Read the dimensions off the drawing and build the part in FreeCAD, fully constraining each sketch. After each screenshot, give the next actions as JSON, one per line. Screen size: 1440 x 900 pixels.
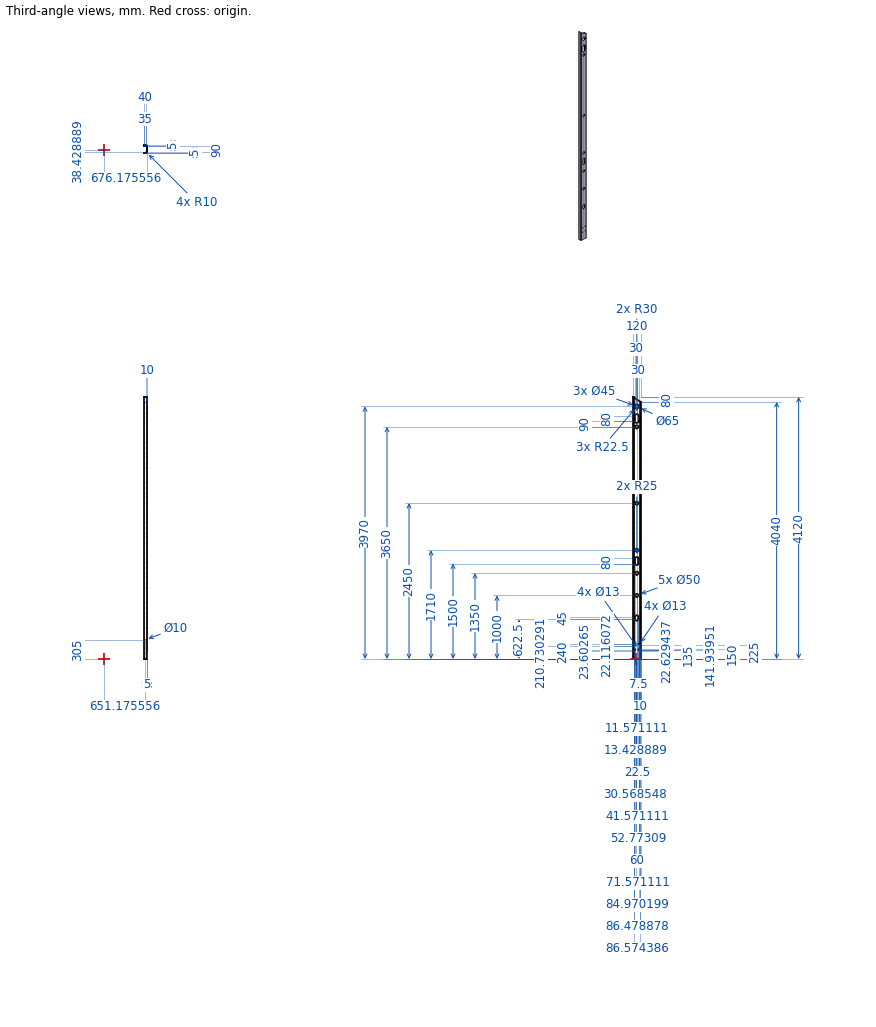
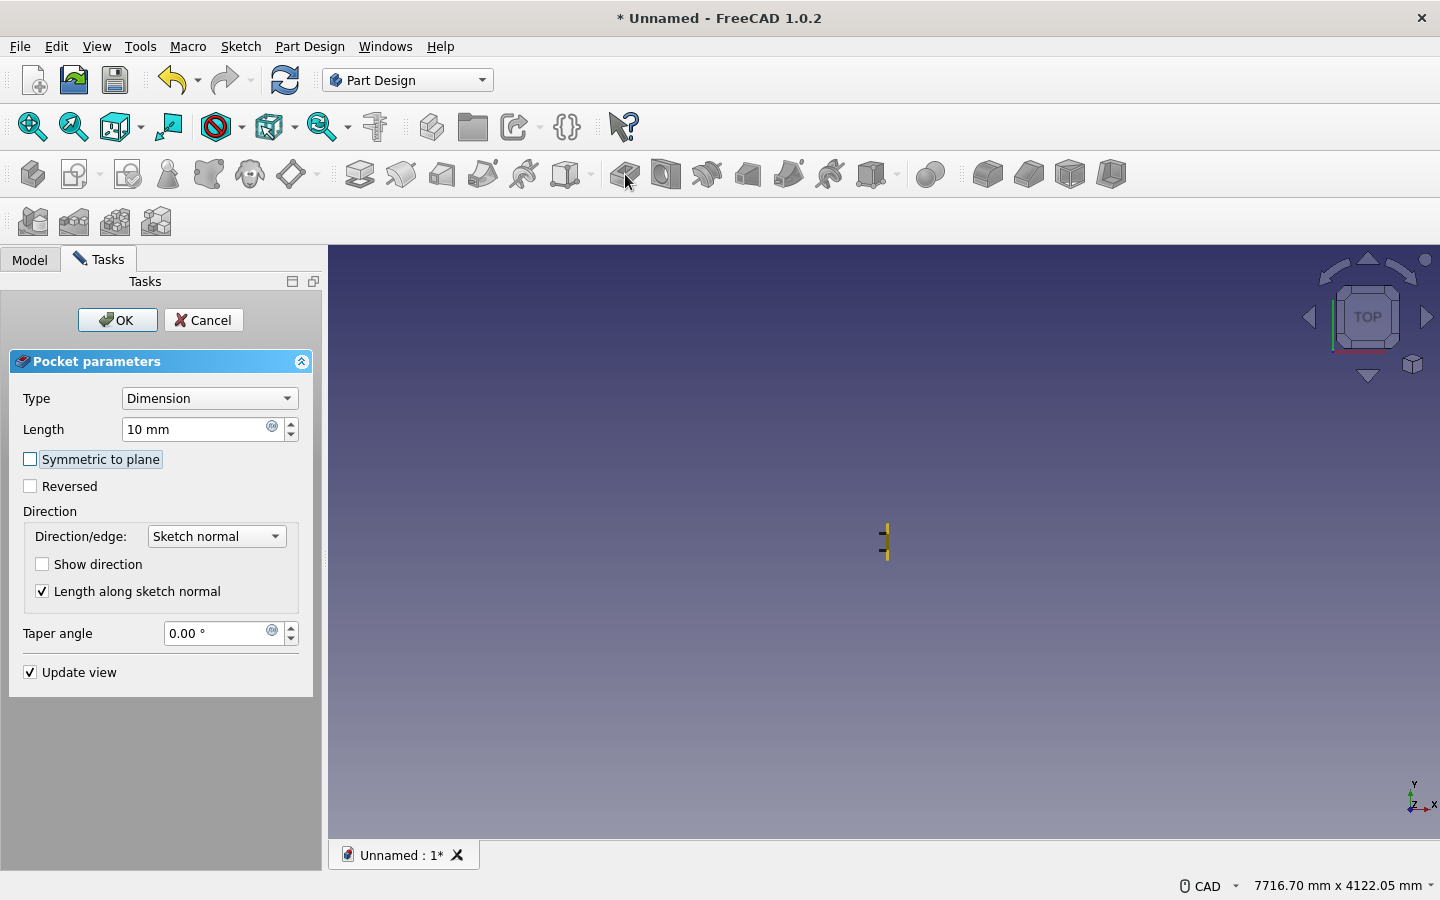
{"action": "left_click", "coordinate": [118, 320]}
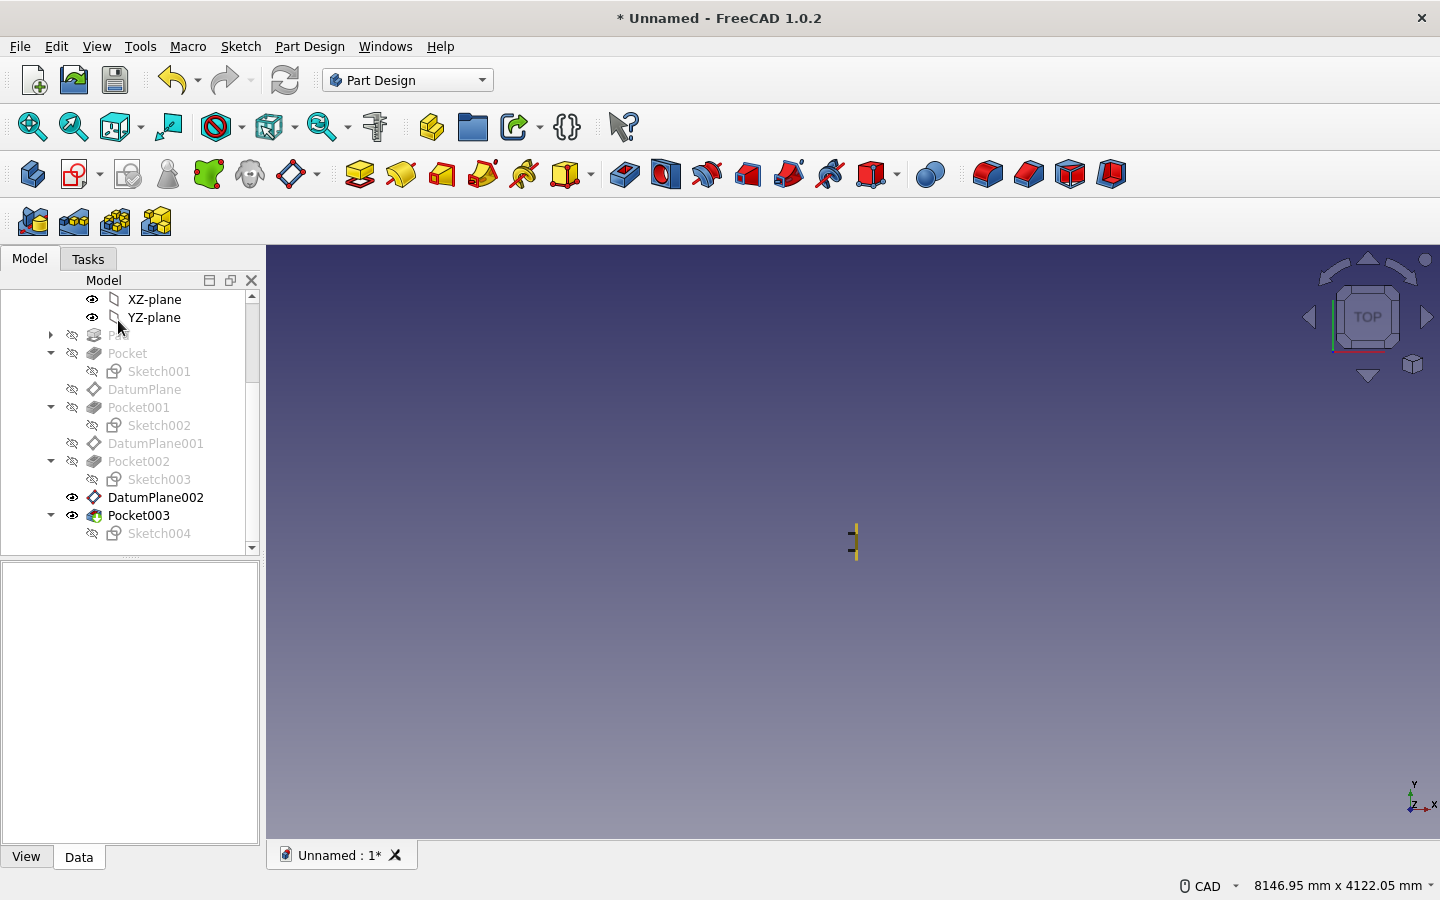
{"action": "left_click", "coordinate": [117, 497]}
{"action": "key", "text": "space"}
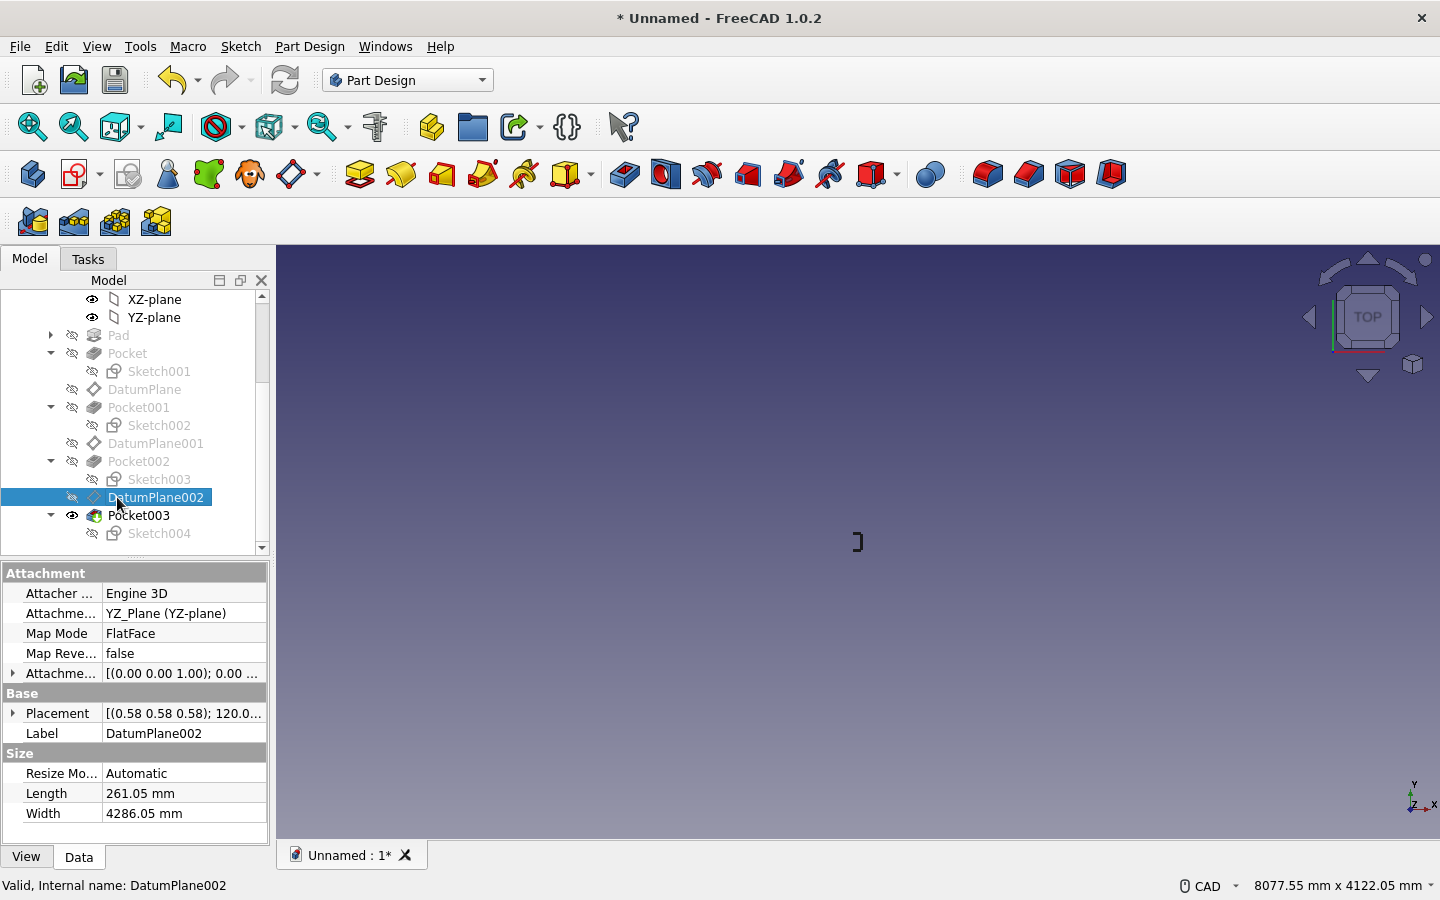
{"action": "left_click", "coordinate": [33, 128]}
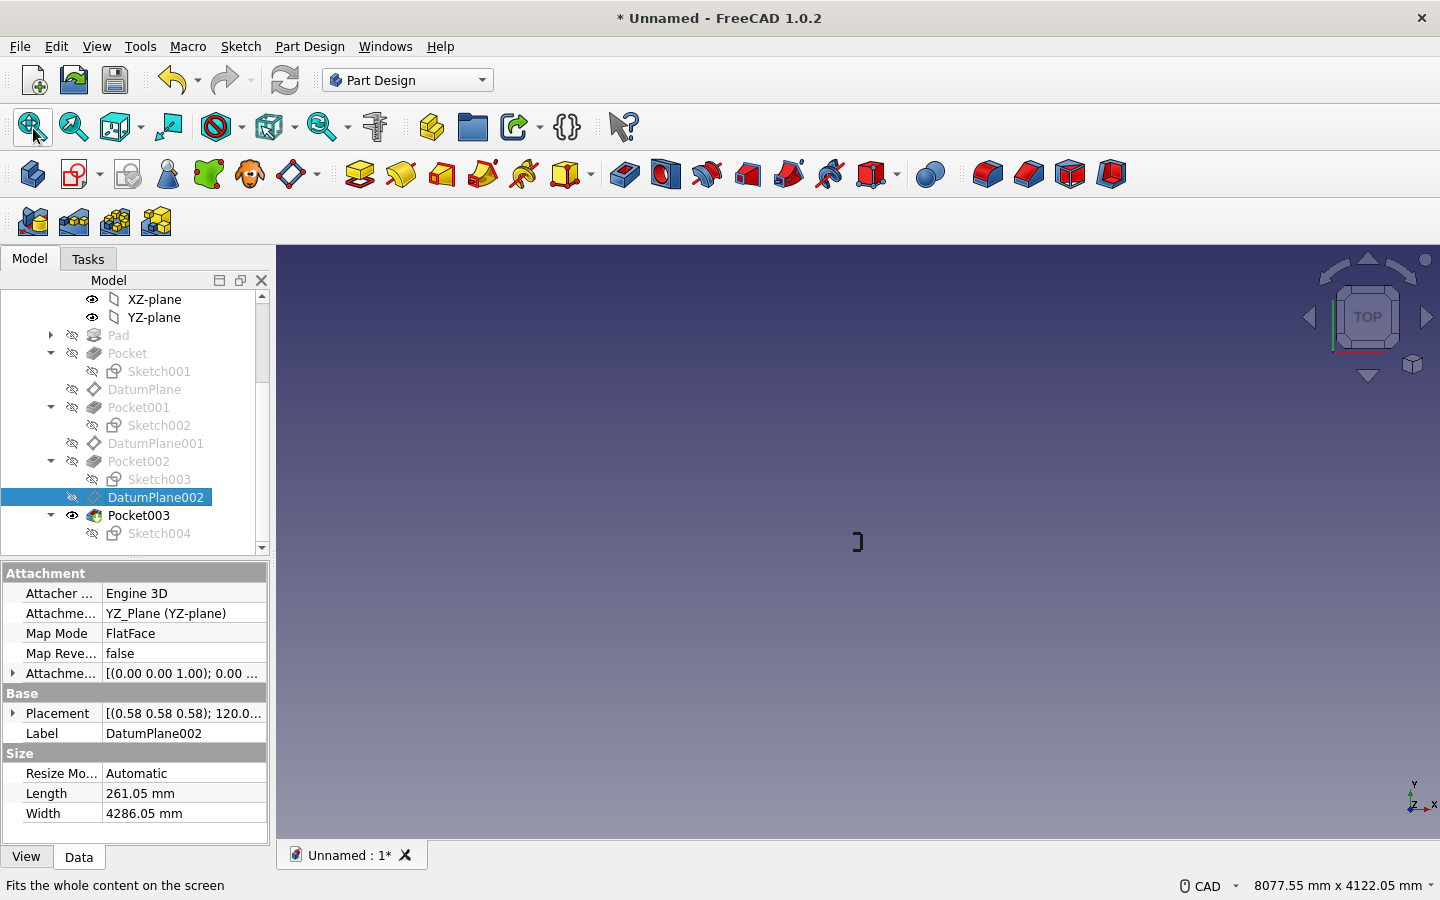
{"action": "key", "text": "0"}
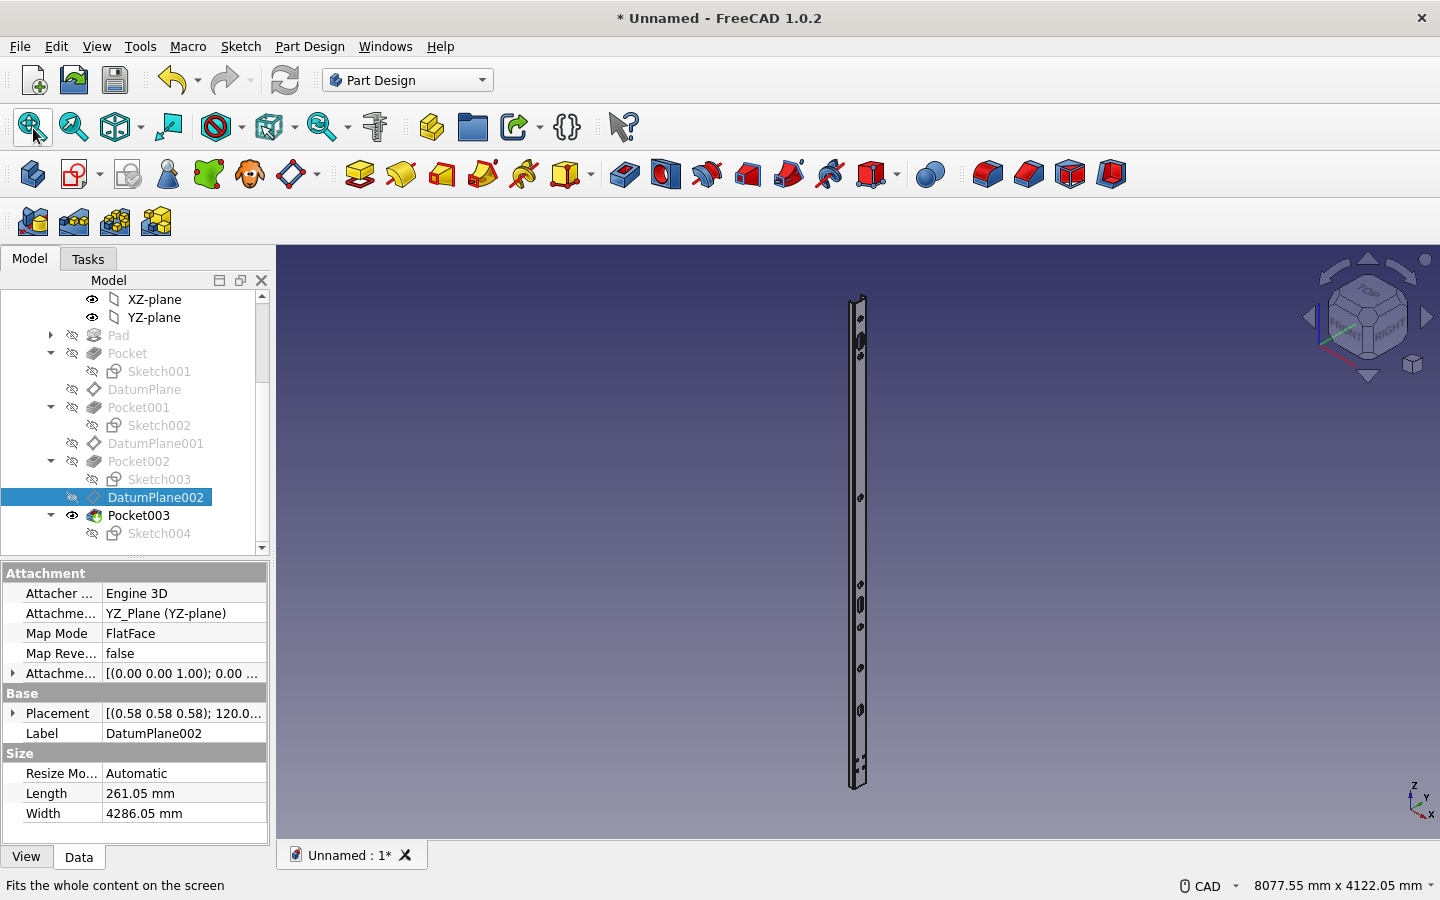
{"action": "key", "text": "3"}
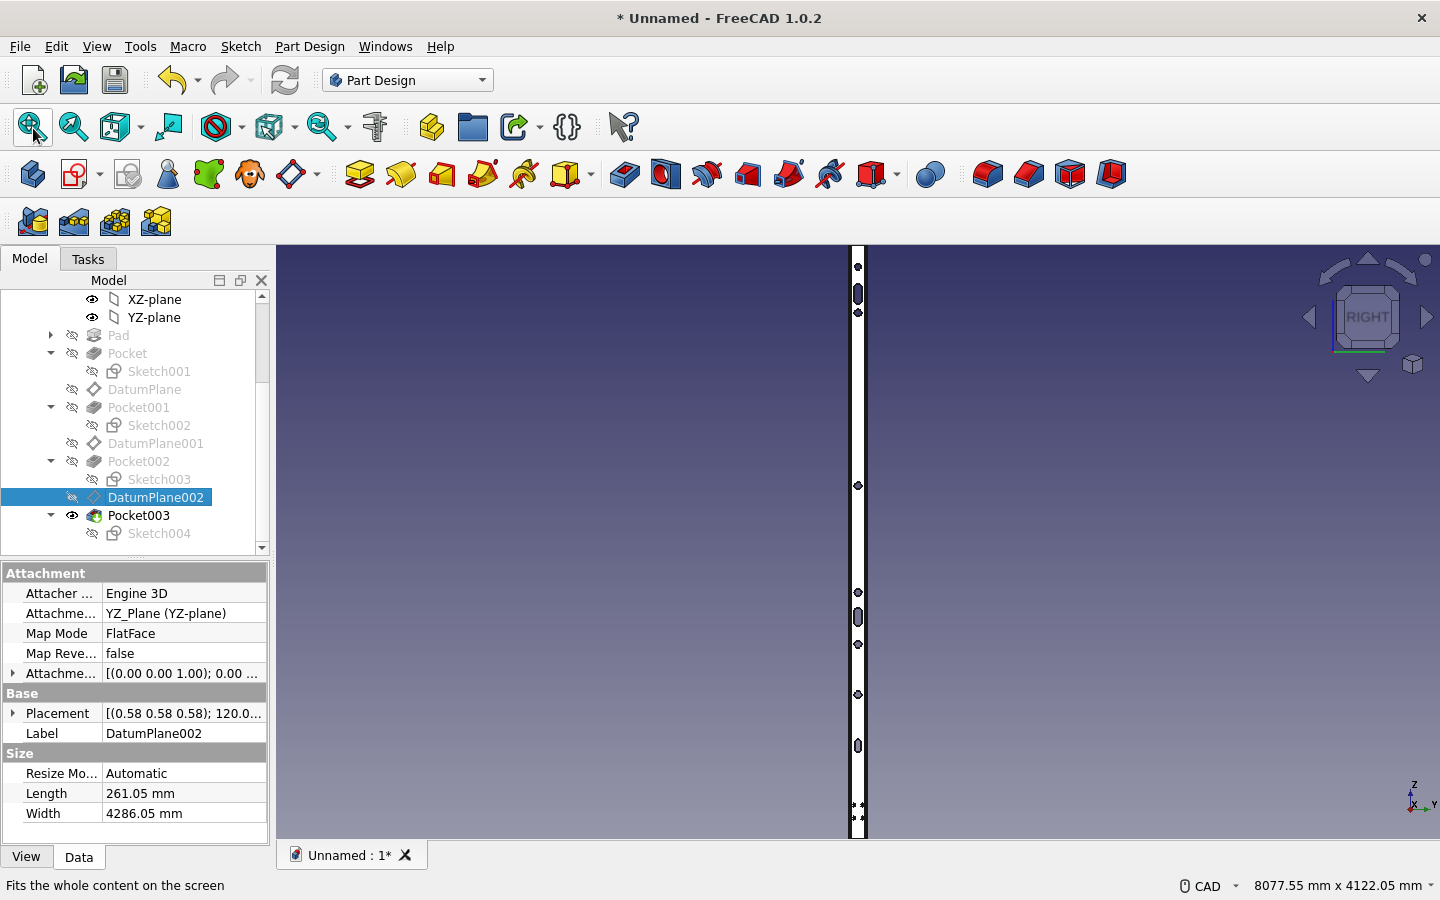
{"action": "key", "text": "v f"}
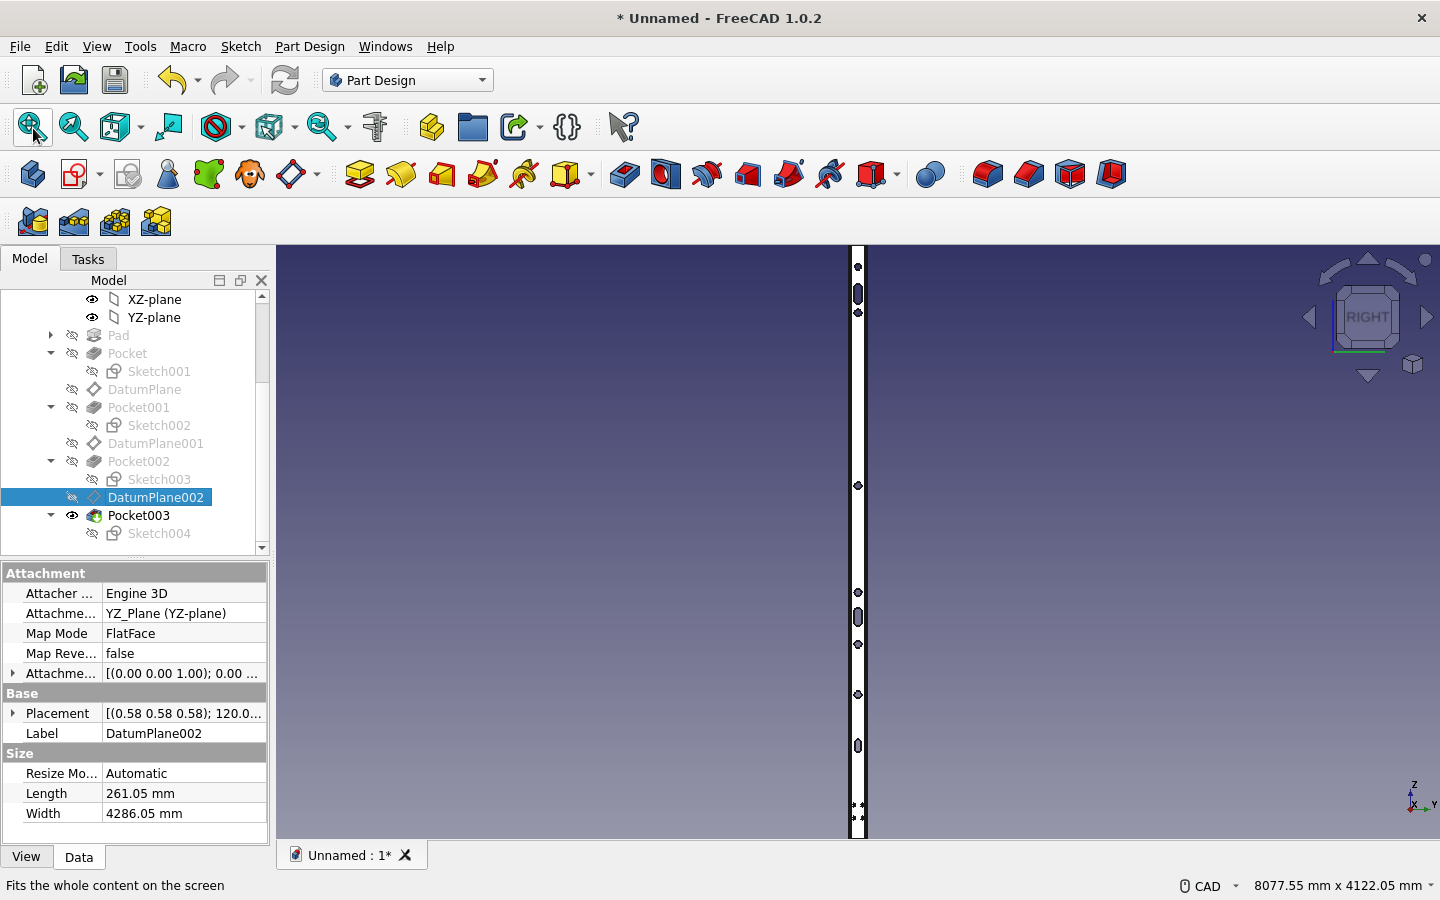
{"action": "key", "text": "2"}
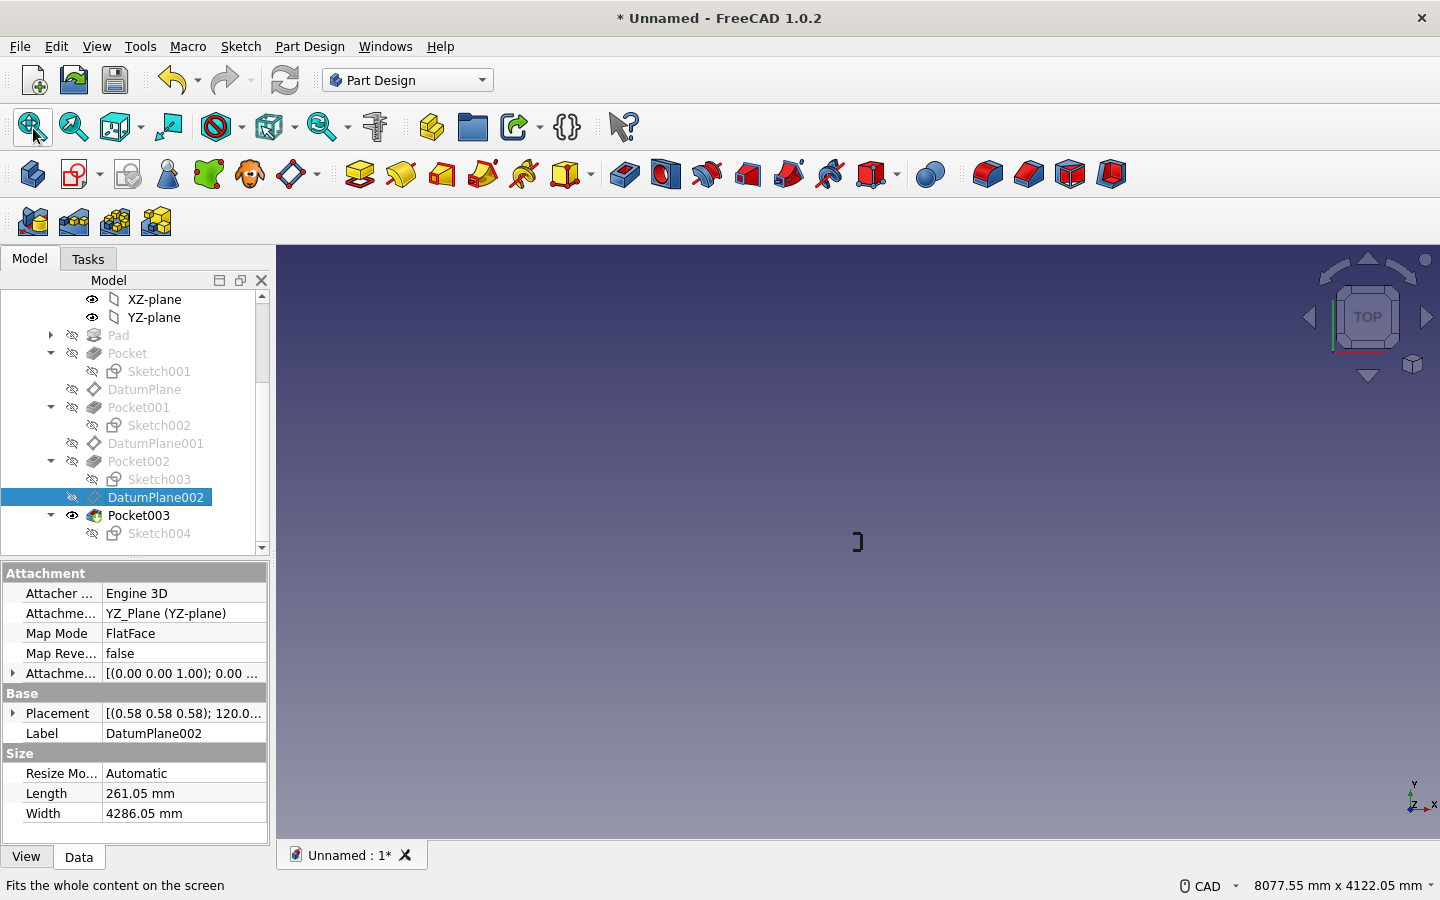
{"action": "key", "text": "v f"}